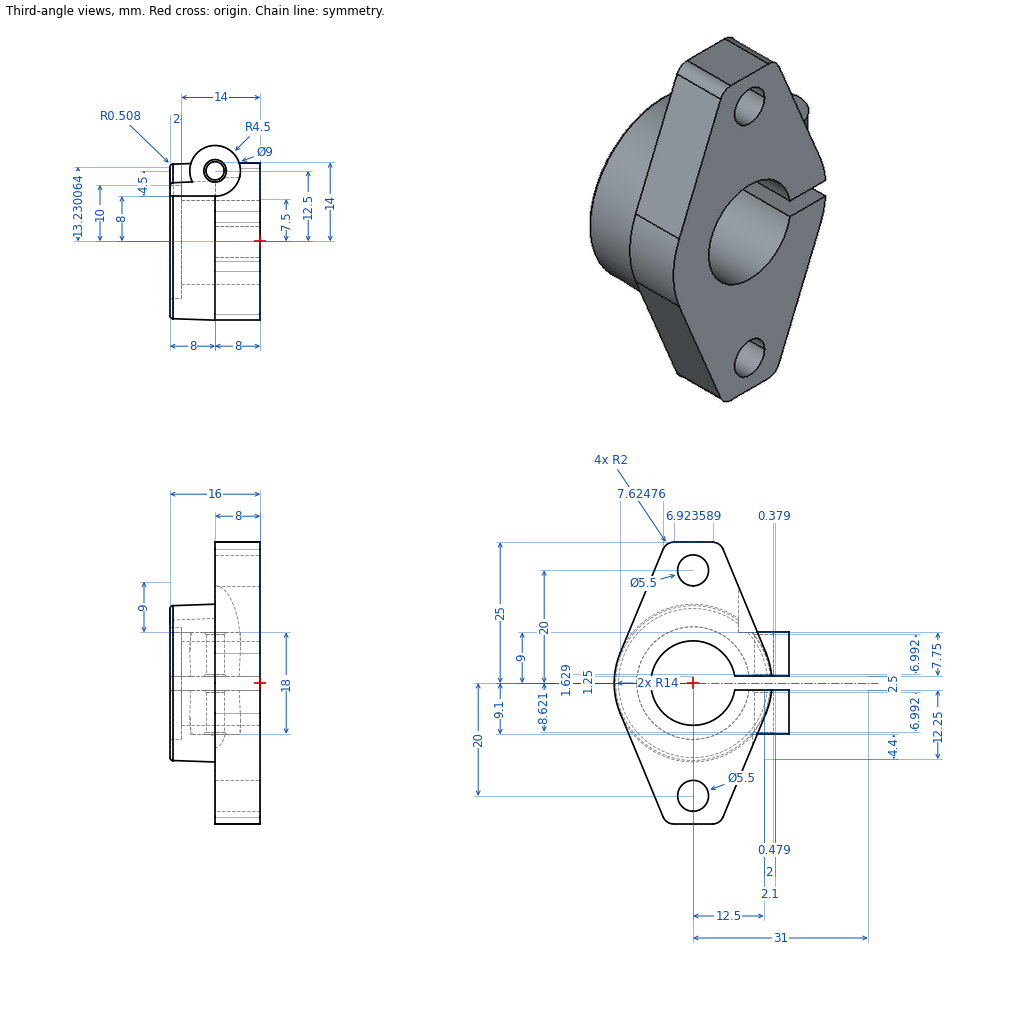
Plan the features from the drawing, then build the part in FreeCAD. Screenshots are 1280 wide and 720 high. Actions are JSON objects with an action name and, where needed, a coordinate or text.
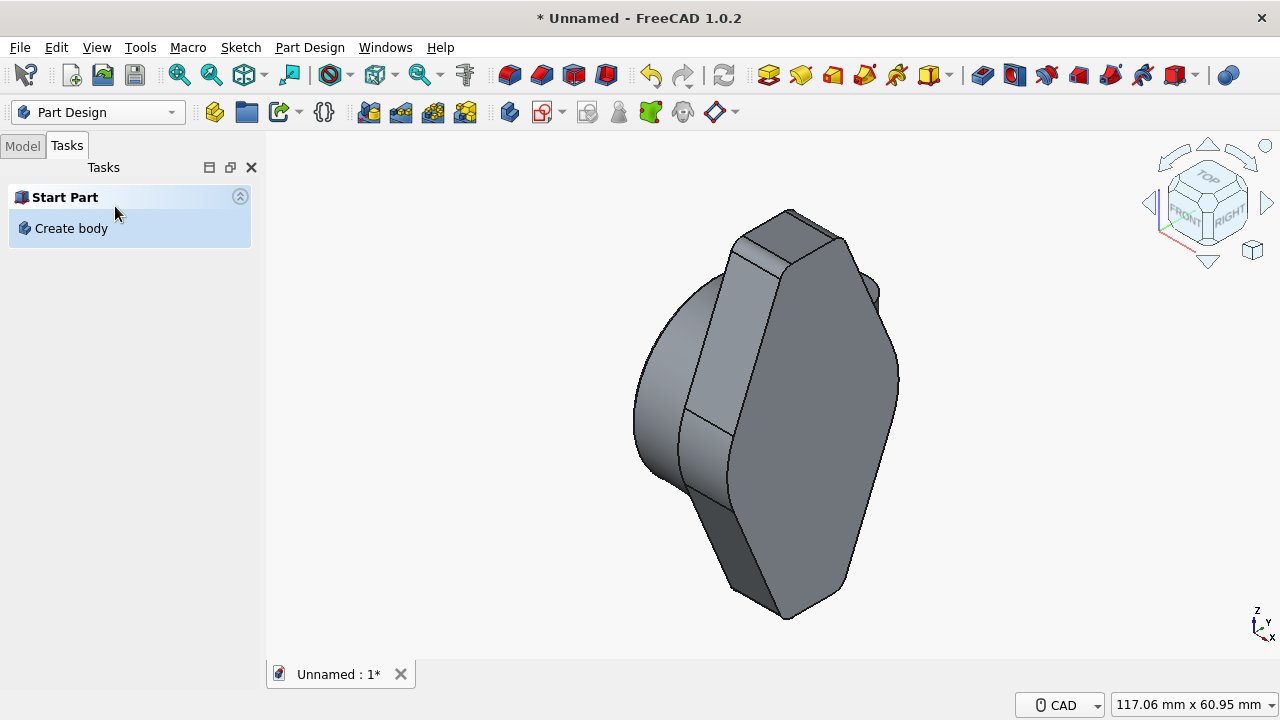
{"action": "left_click", "coordinate": [813, 428]}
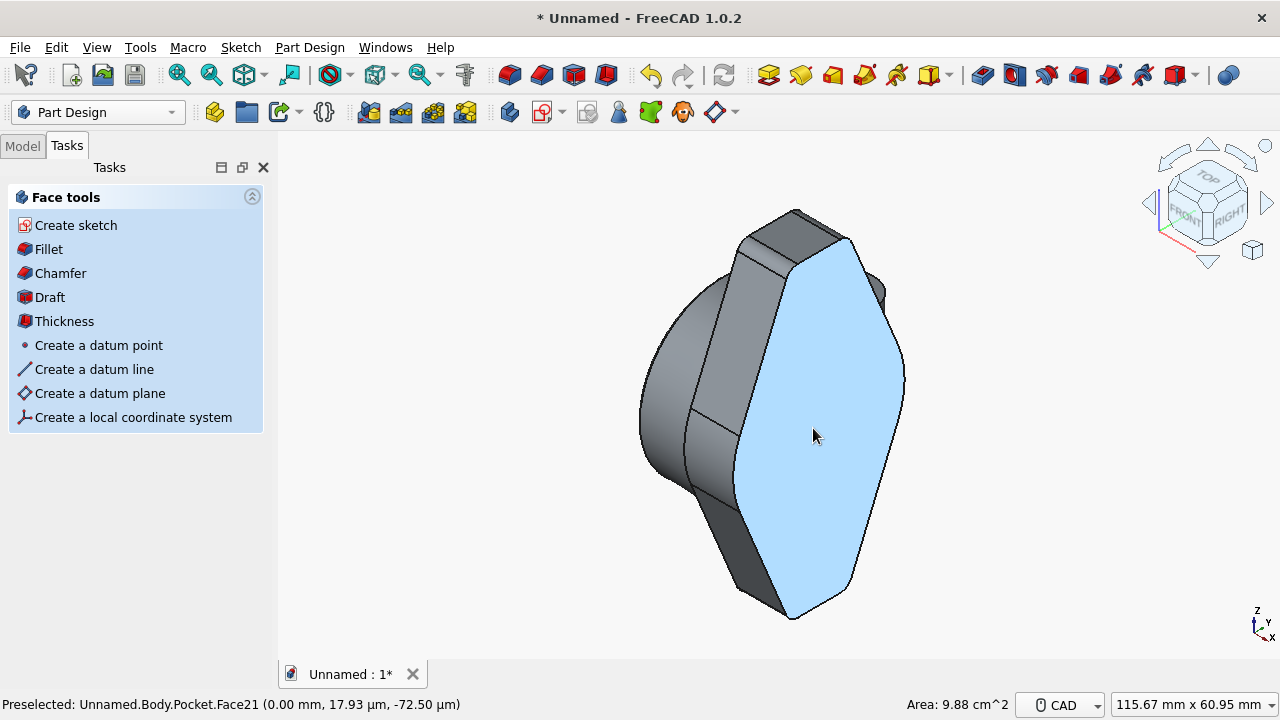
{"action": "left_click", "coordinate": [542, 112]}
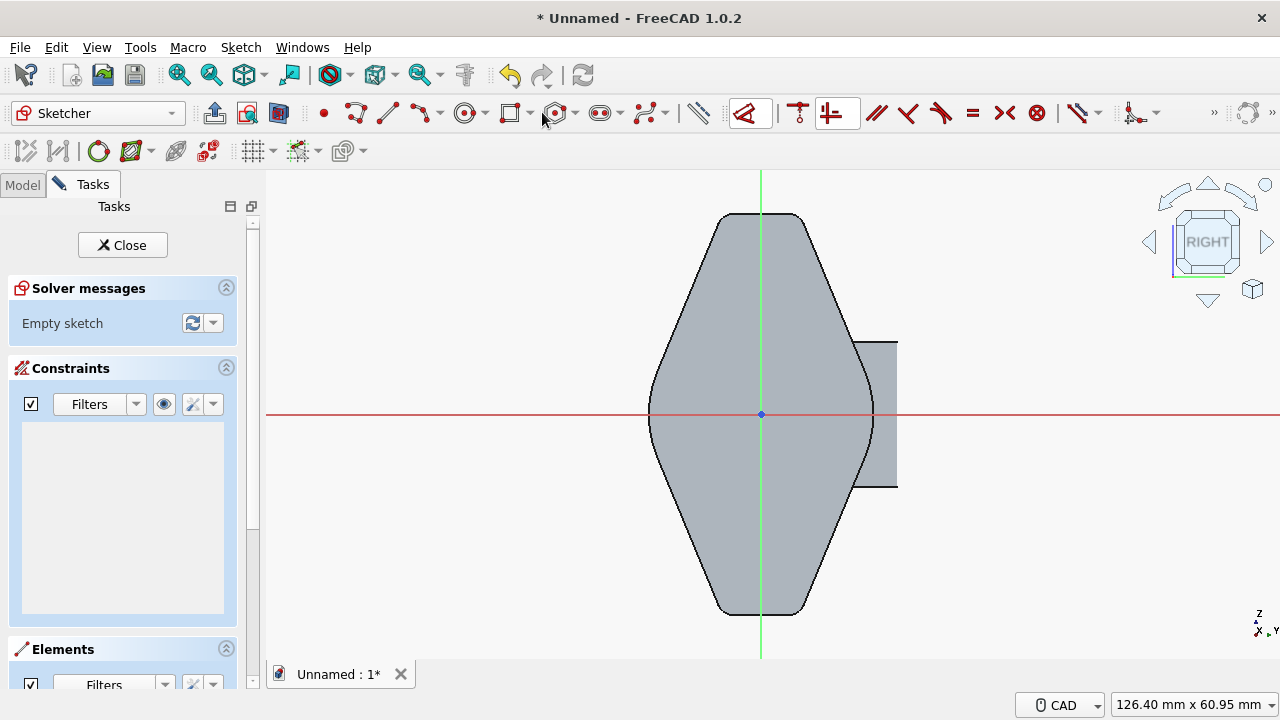
{"action": "scroll", "coordinate": [1033, 414], "scroll_direction": "up", "scroll_amount": 4}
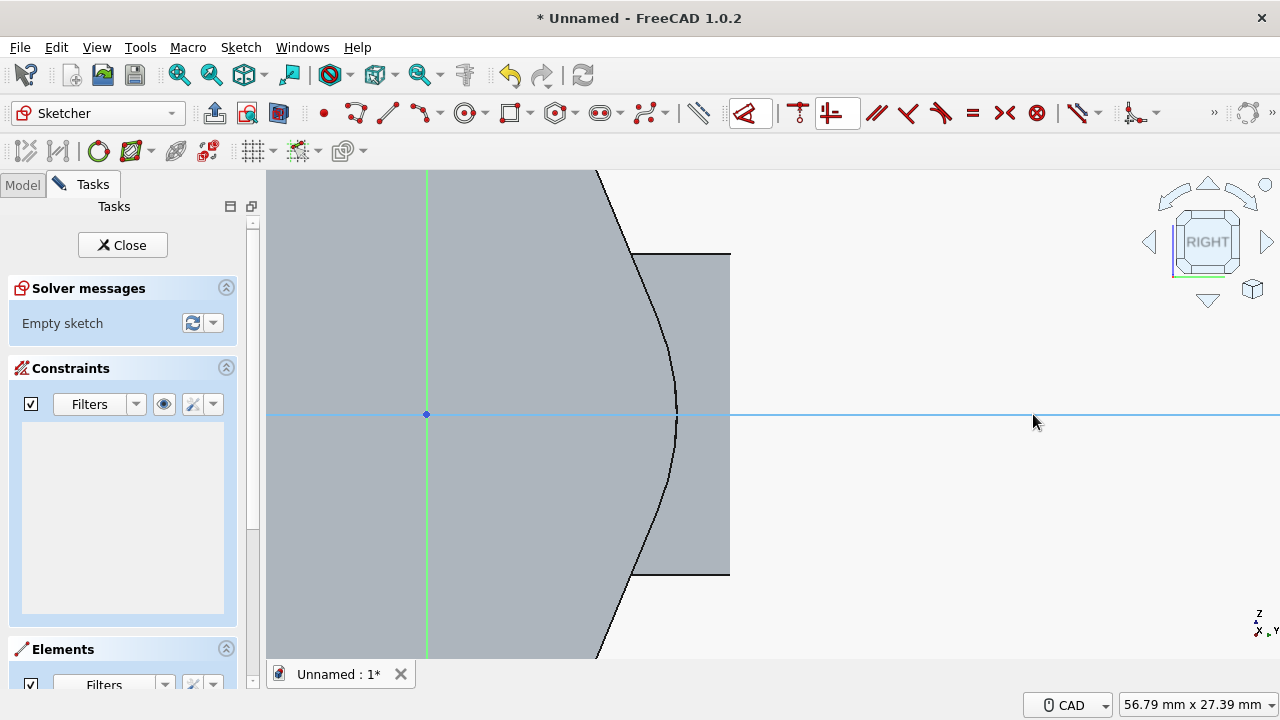
{"action": "left_click", "coordinate": [510, 114]}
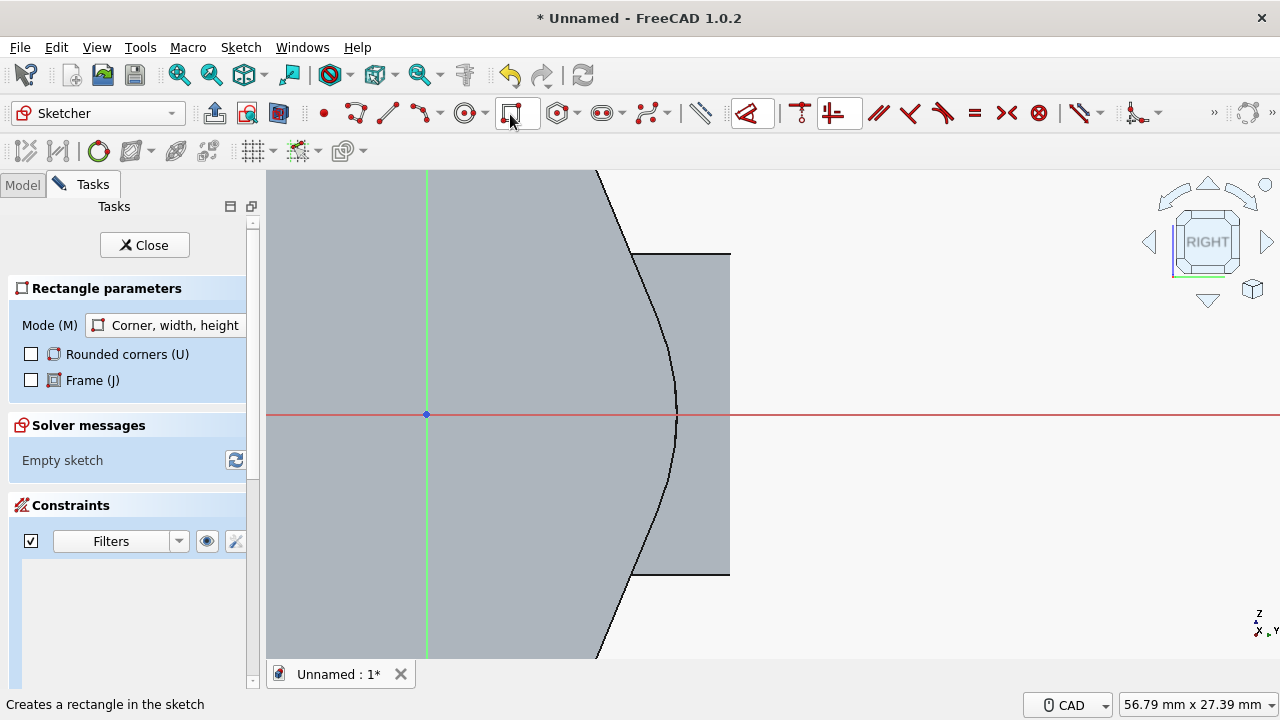
{"action": "left_click", "coordinate": [427, 392]}
{"action": "mouse_move", "coordinate": [980, 437]}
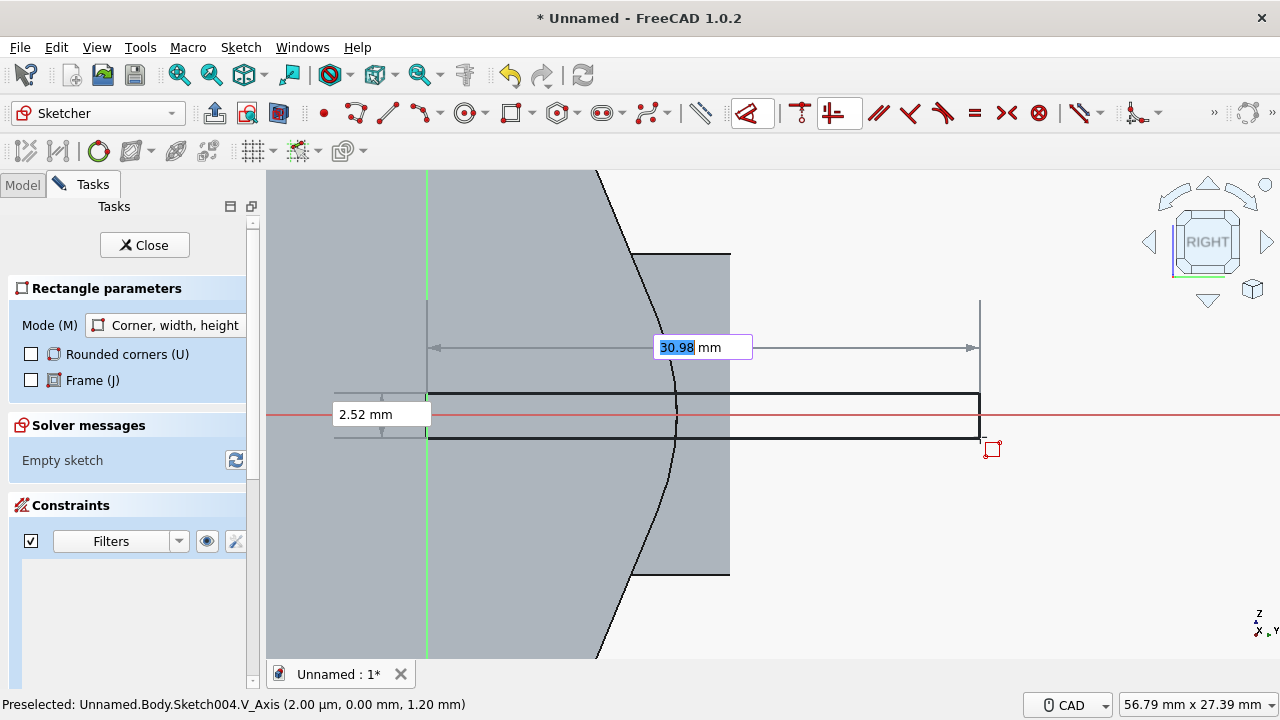
{"action": "type", "text": "31"}
{"action": "key", "text": "Tab"}
{"action": "type", "text": "2.5"}
{"action": "key", "text": "Return"}
{"action": "key", "text": "Escape"}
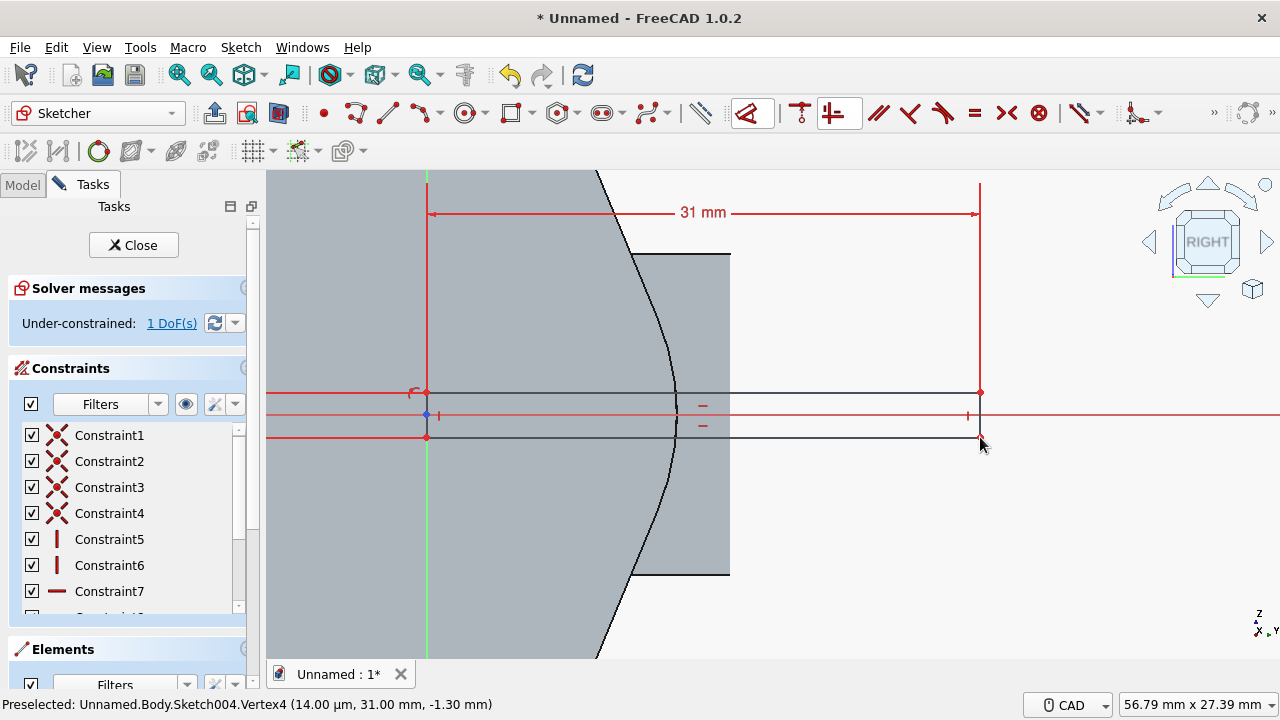
{"action": "scroll", "coordinate": [427, 393], "scroll_direction": "up", "scroll_amount": 3}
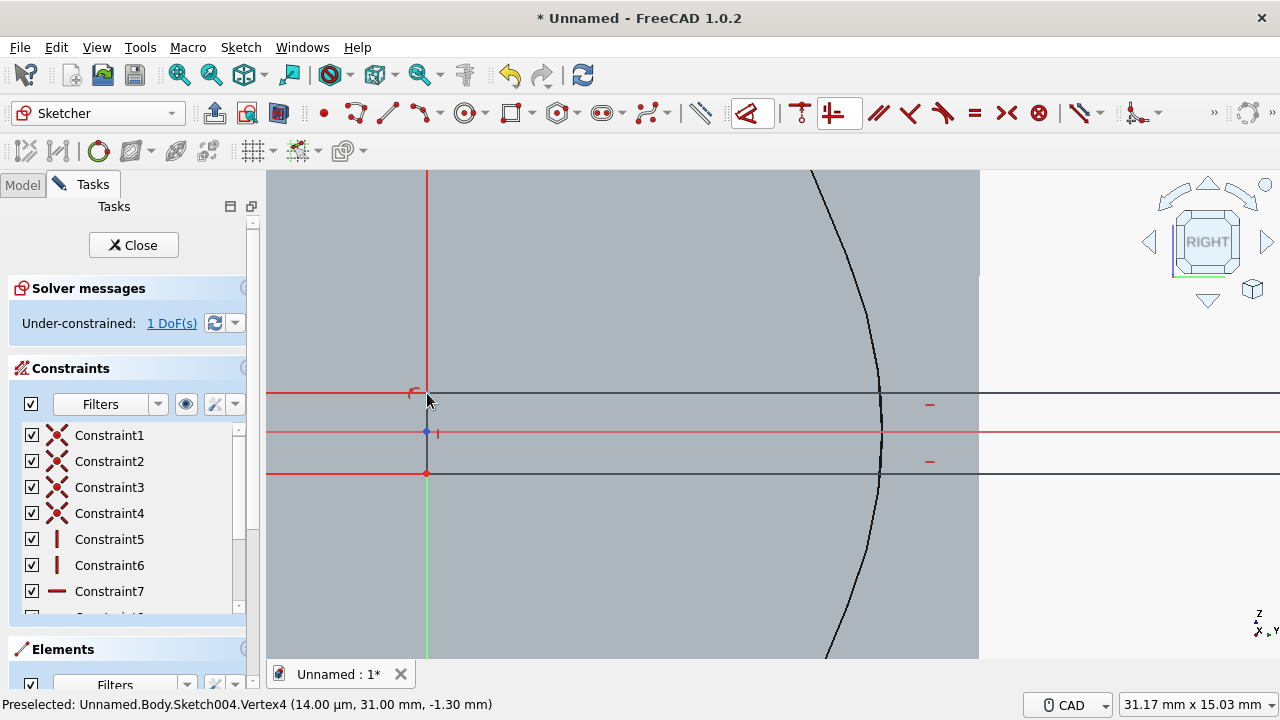
{"action": "left_click", "coordinate": [427, 393]}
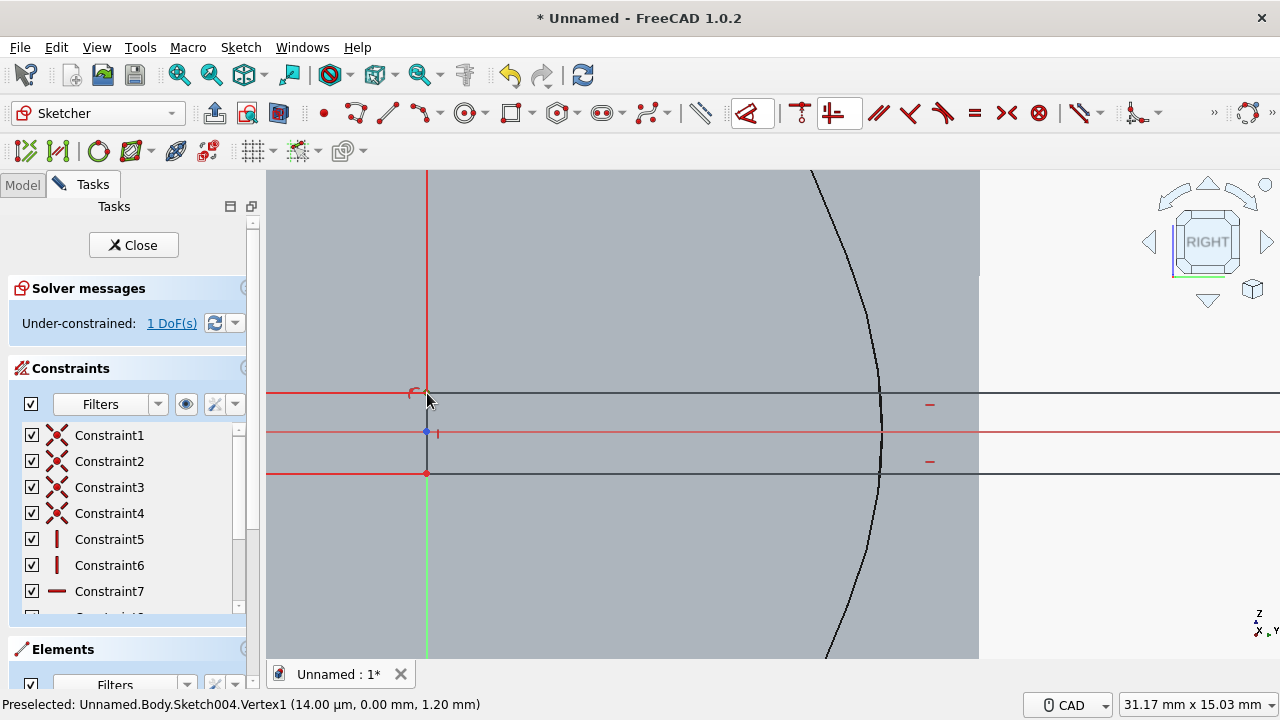
{"action": "left_click", "coordinate": [768, 114]}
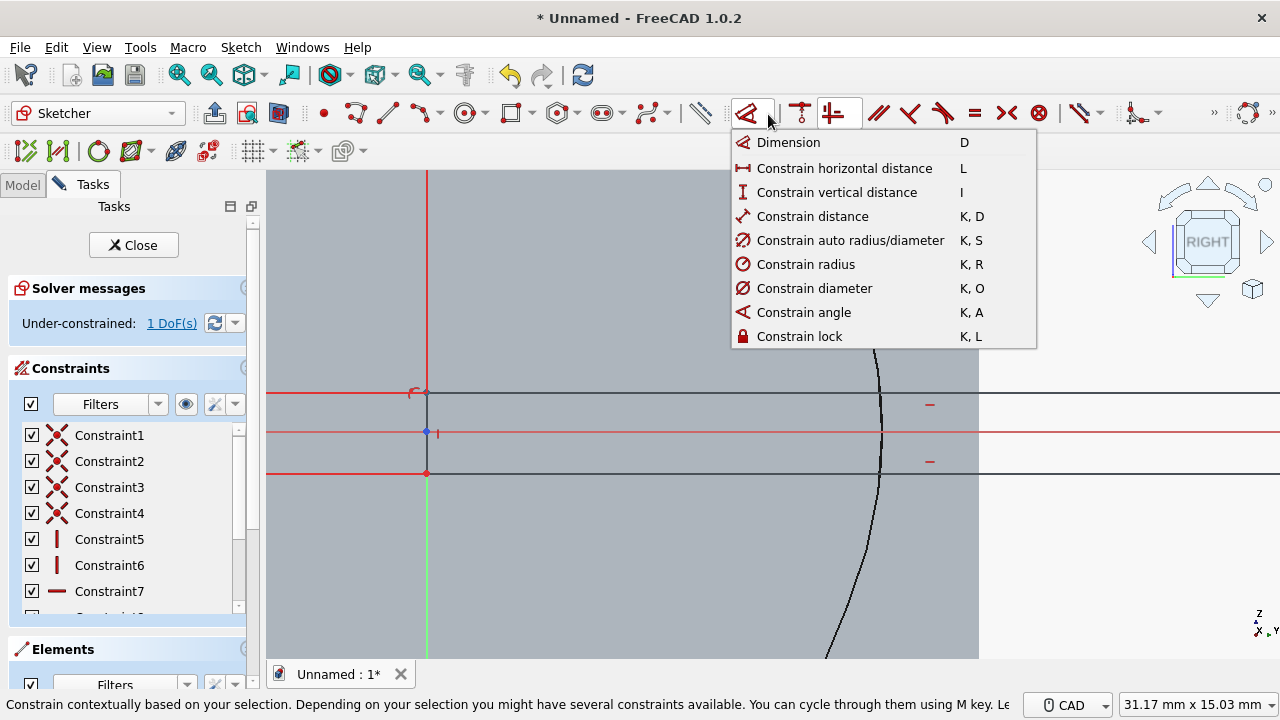
{"action": "left_click", "coordinate": [884, 192]}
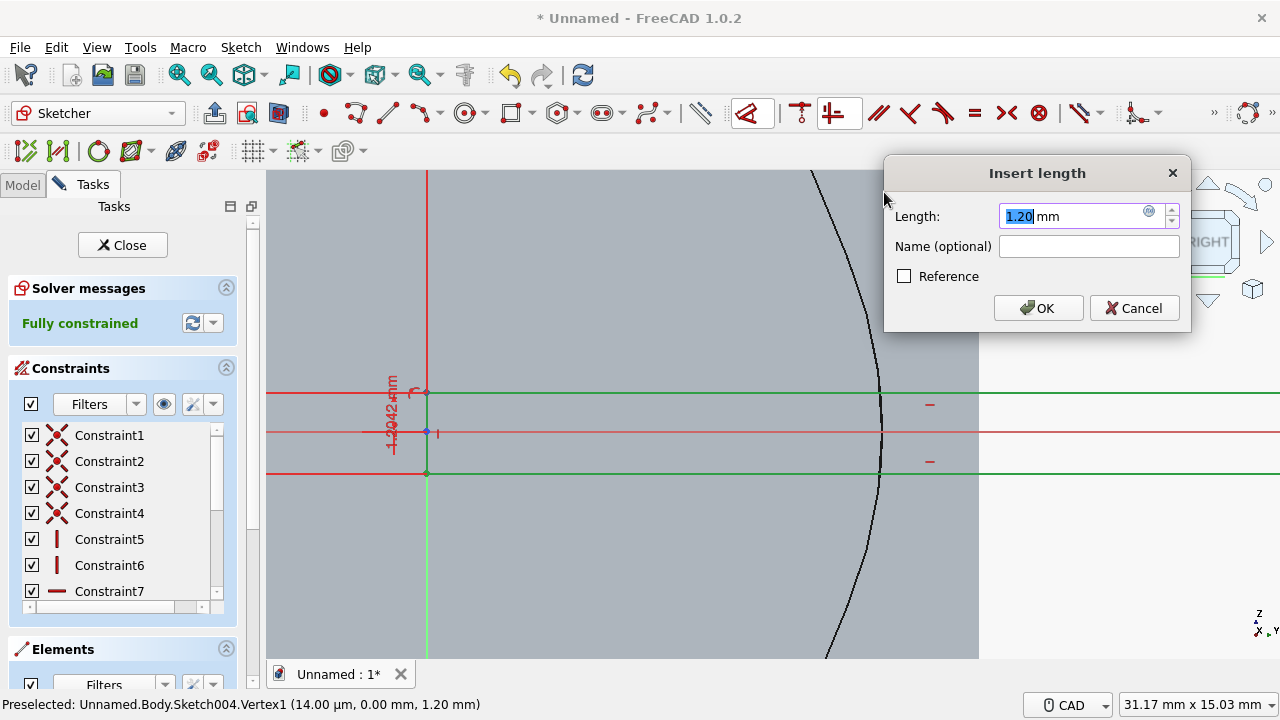
{"action": "type", "text": "1.25"}
{"action": "key", "text": "Return"}